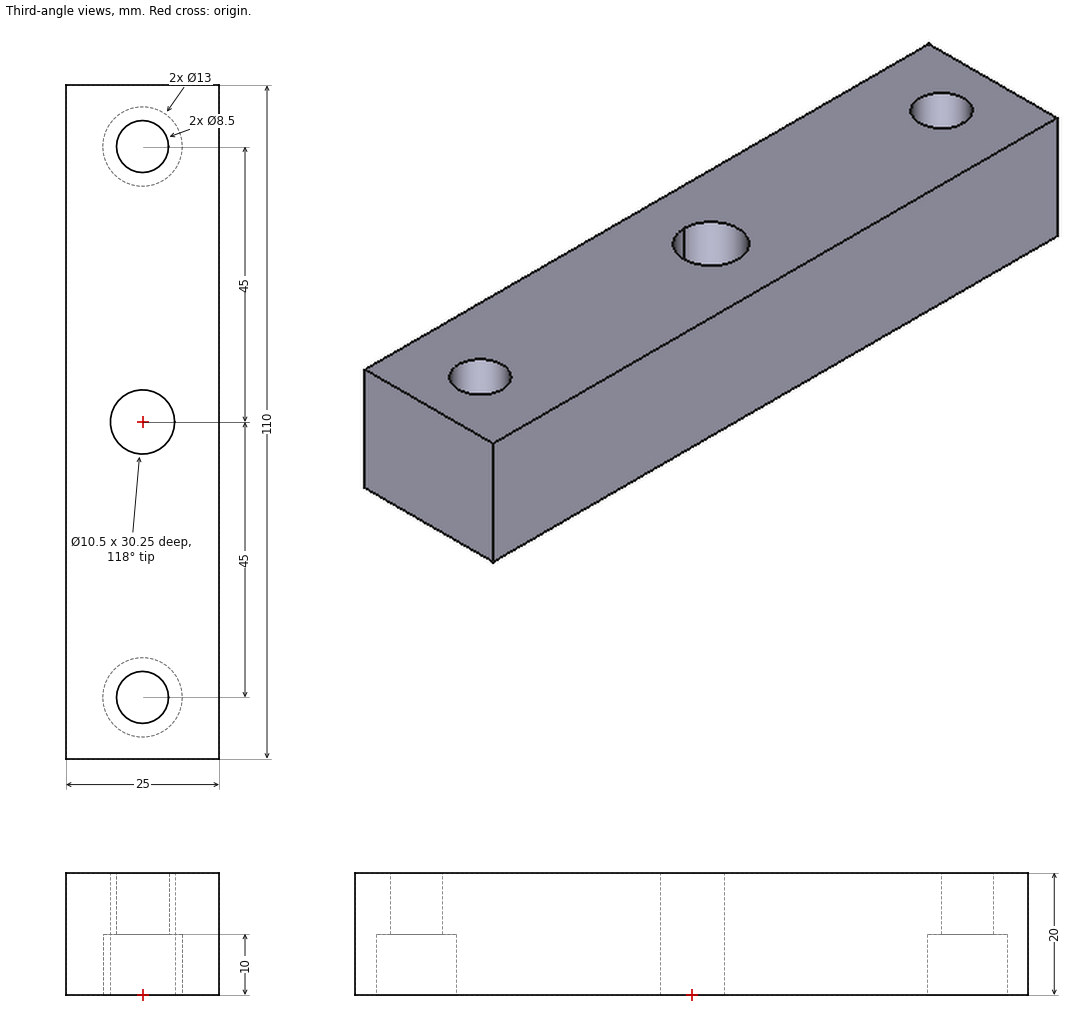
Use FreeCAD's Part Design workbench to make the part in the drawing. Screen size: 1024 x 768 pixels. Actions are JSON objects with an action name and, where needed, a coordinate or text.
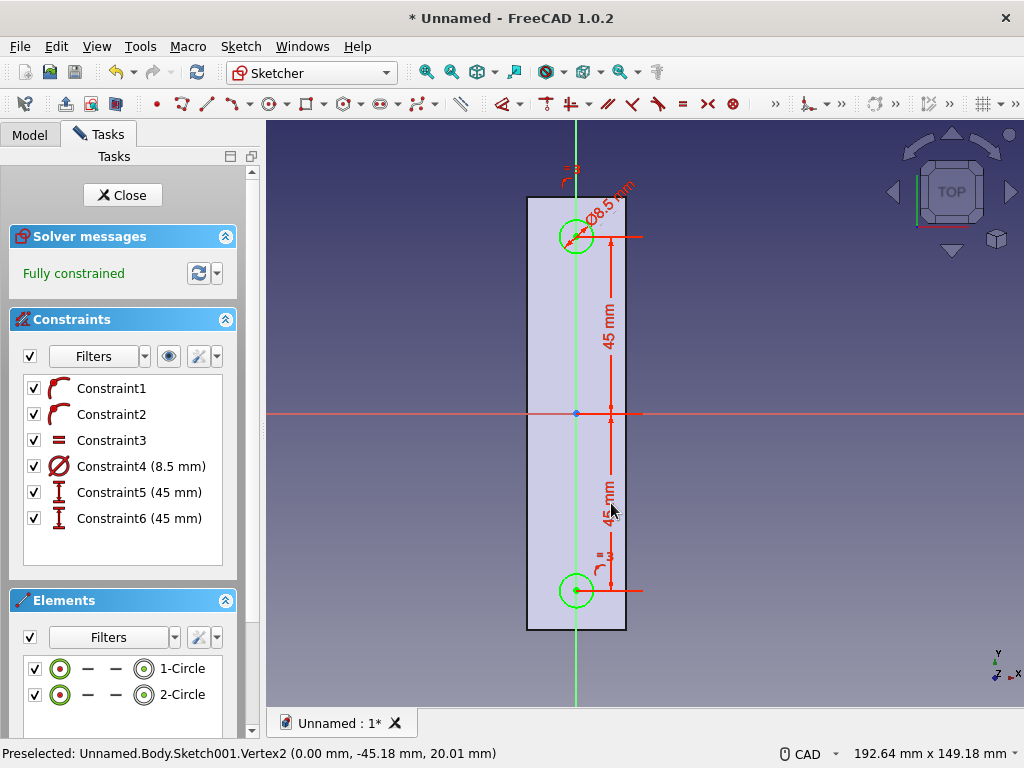
{"action": "left_click", "coordinate": [123, 195]}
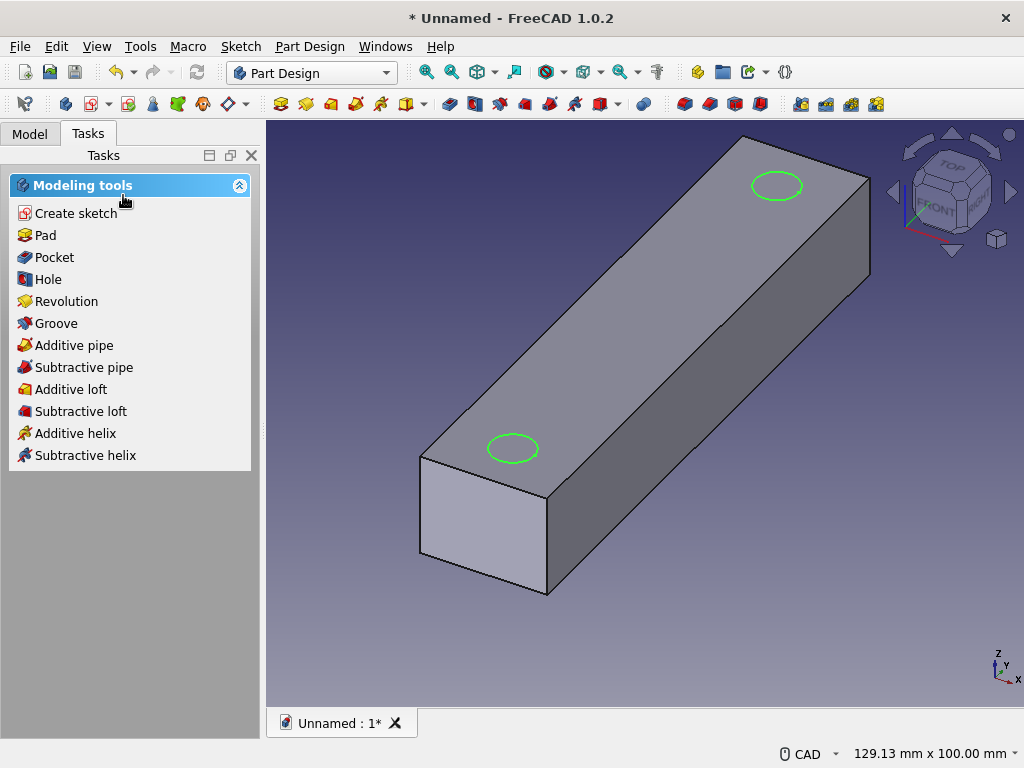
{"action": "left_click", "coordinate": [450, 104]}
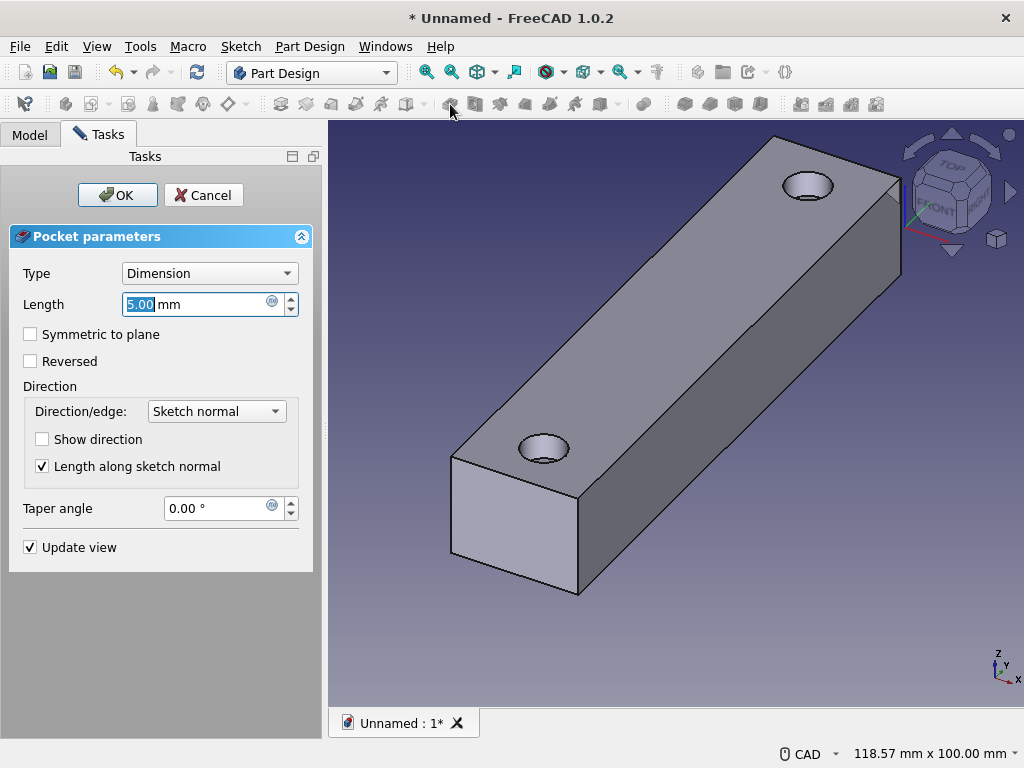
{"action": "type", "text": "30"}
{"action": "key", "text": "Tab"}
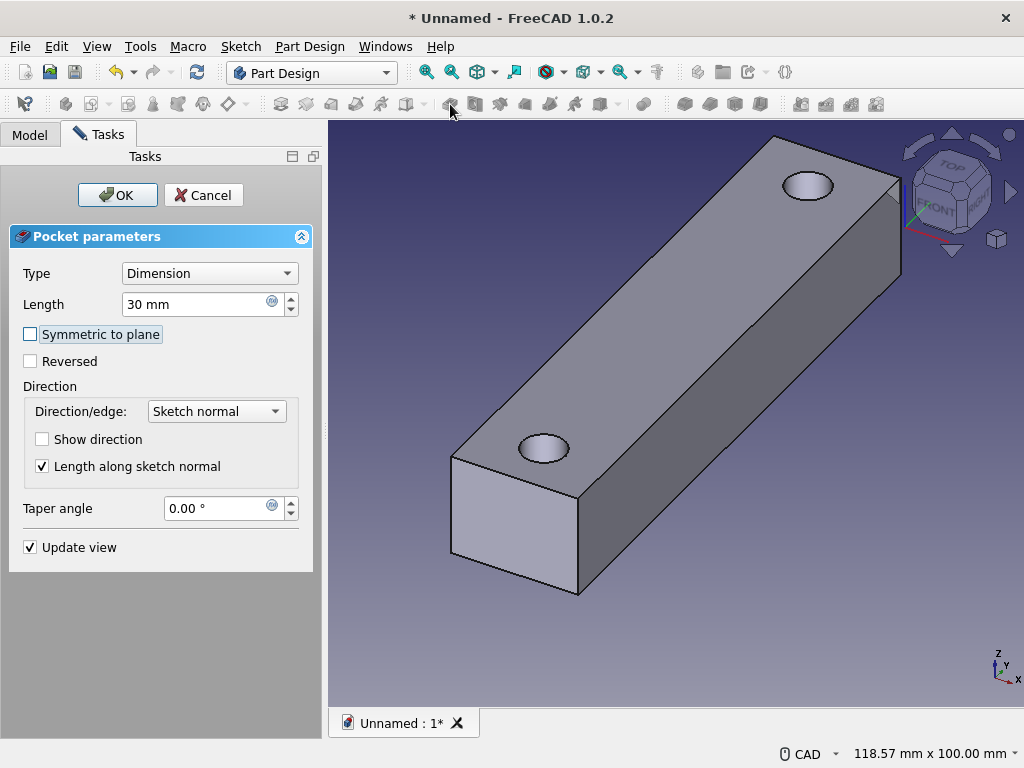
{"action": "left_click", "coordinate": [118, 195]}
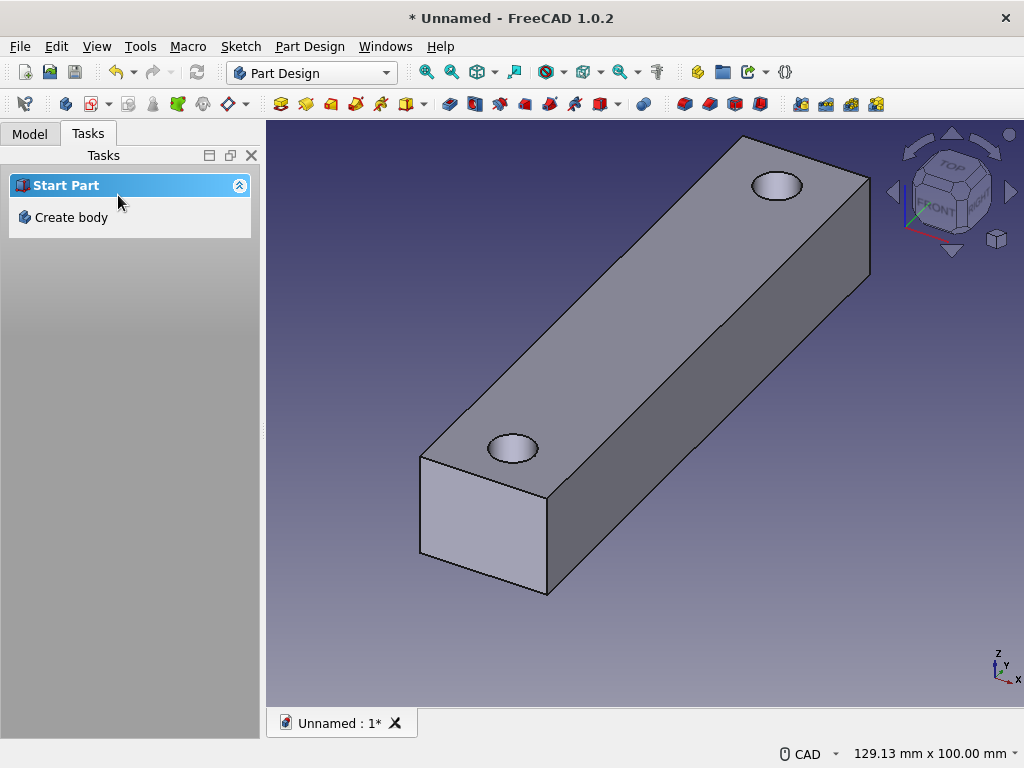
{"action": "key", "text": "5"}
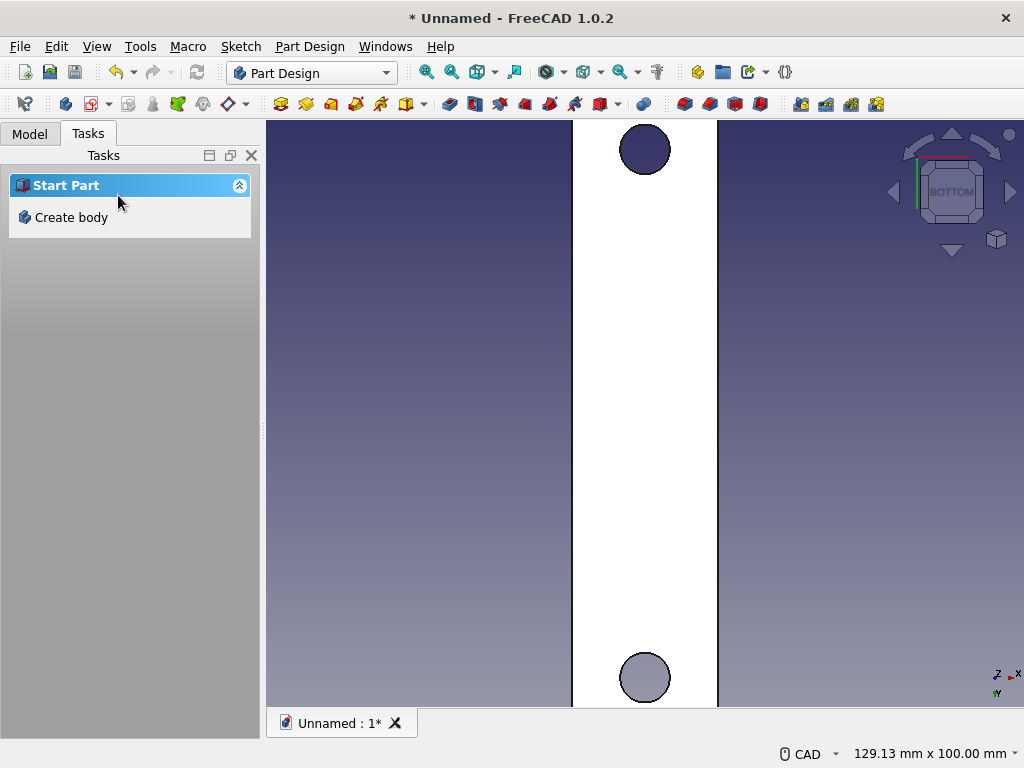
{"action": "left_click", "coordinate": [427, 72]}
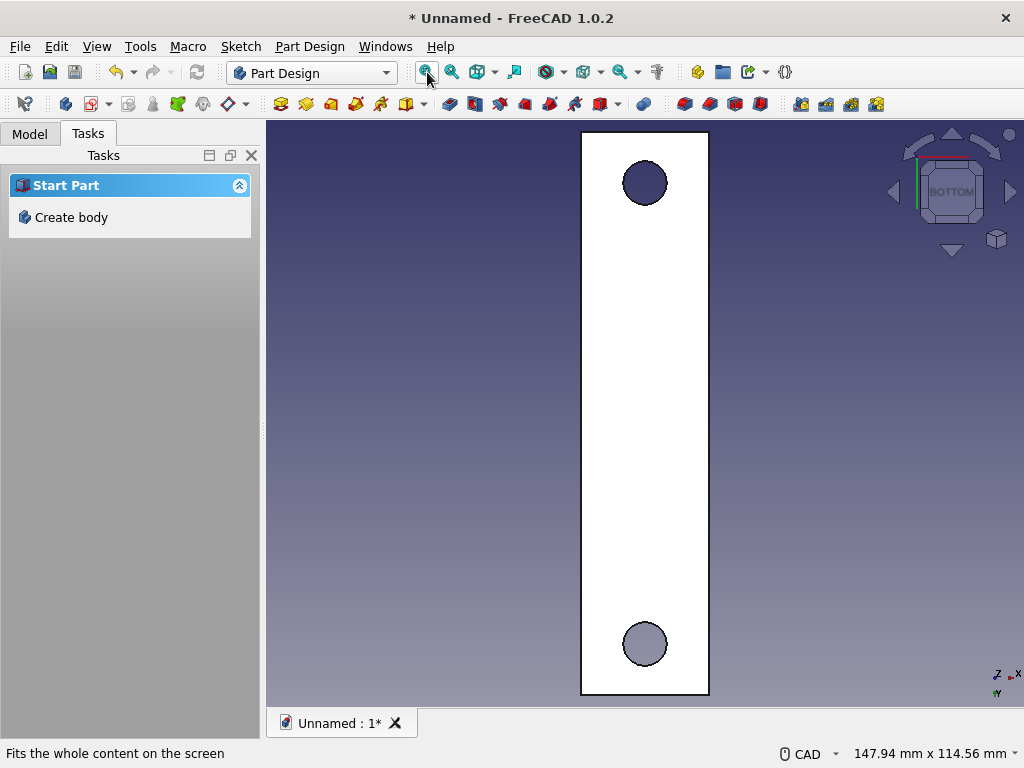
{"action": "left_click", "coordinate": [645, 493]}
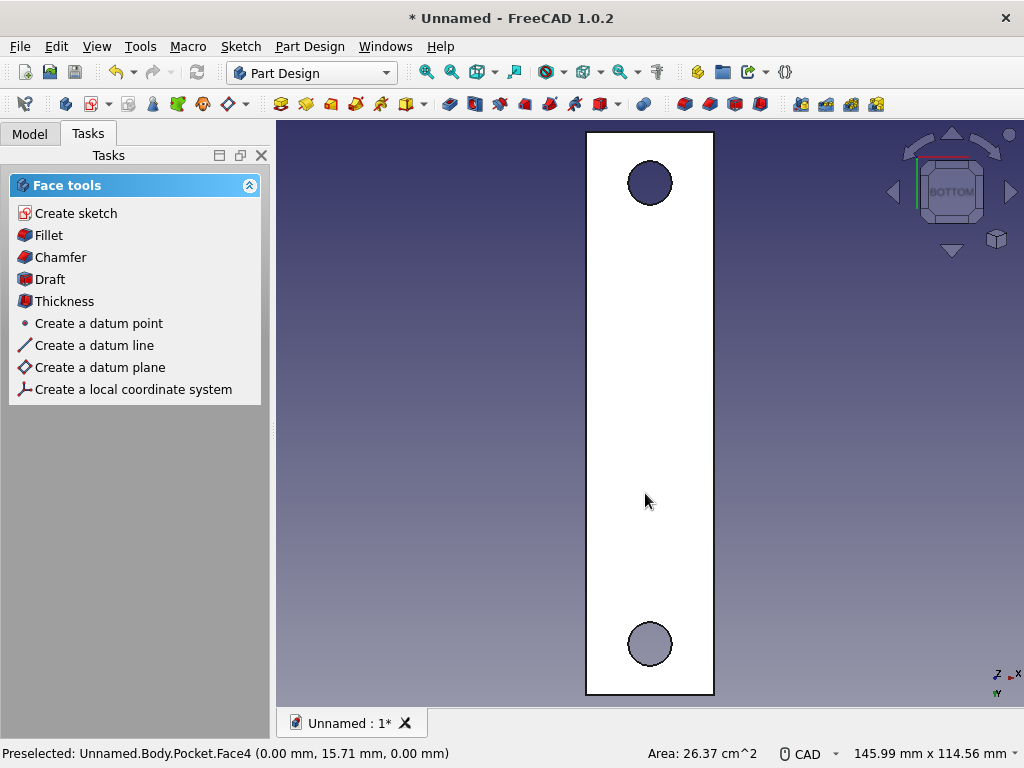
{"action": "left_click", "coordinate": [90, 104]}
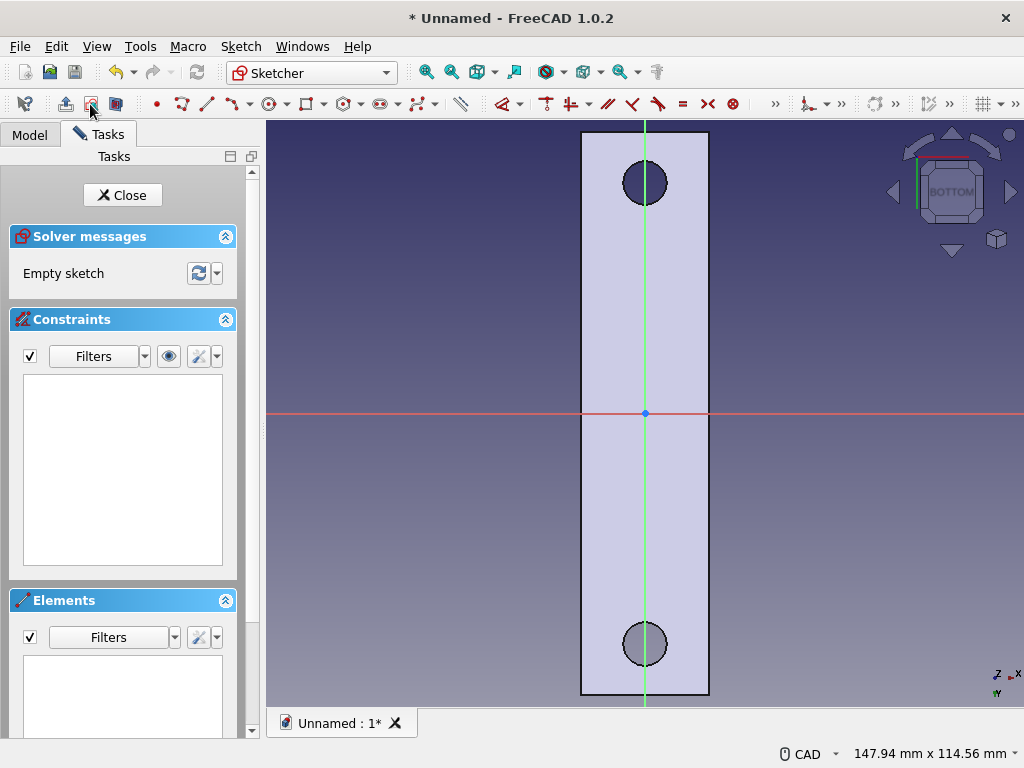
{"action": "scroll", "coordinate": [437, 414], "scroll_direction": "down", "scroll_amount": 2}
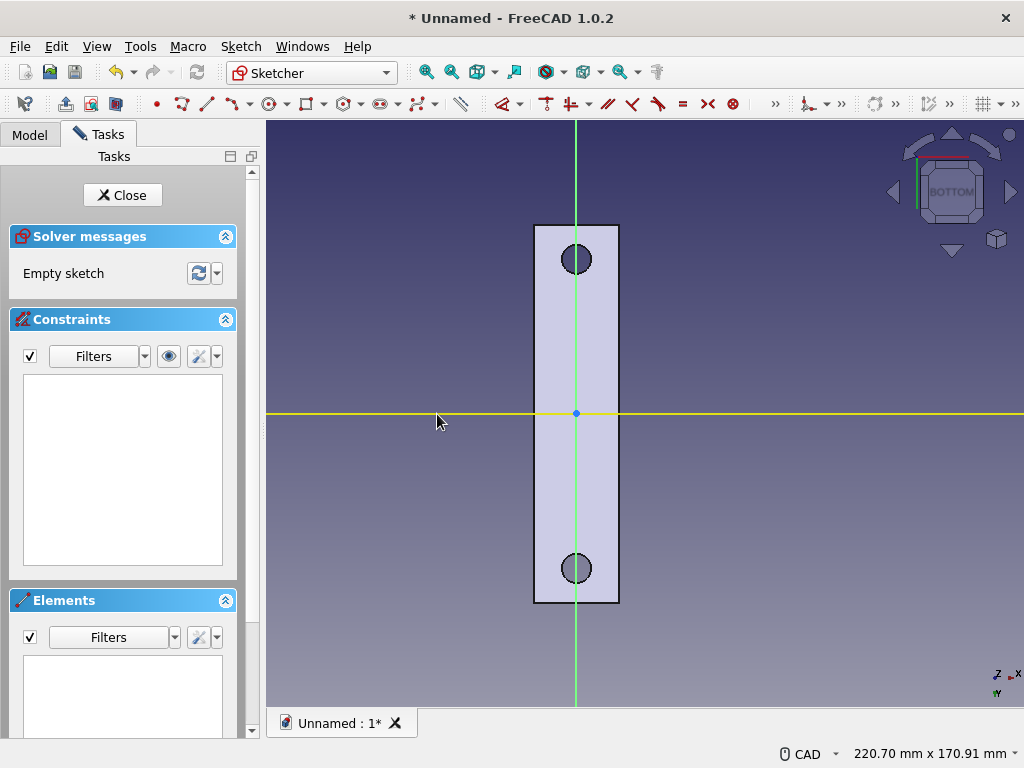
{"action": "key", "text": "g c"}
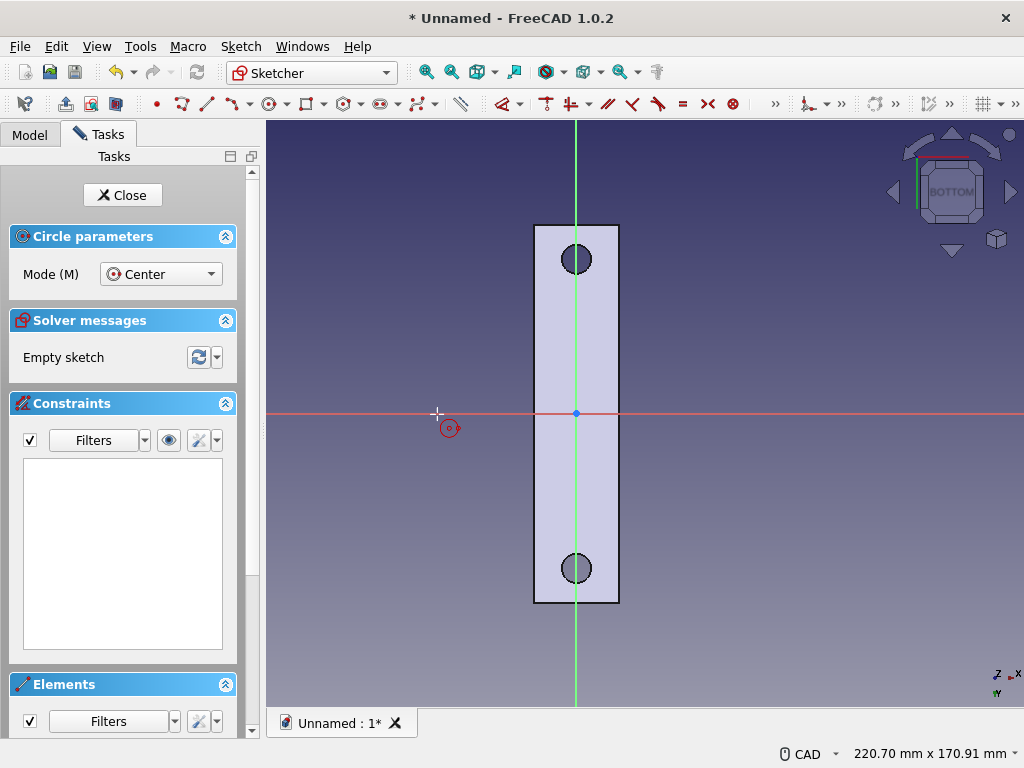
{"action": "left_click", "coordinate": [577, 568]}
{"action": "left_click", "coordinate": [592, 553]}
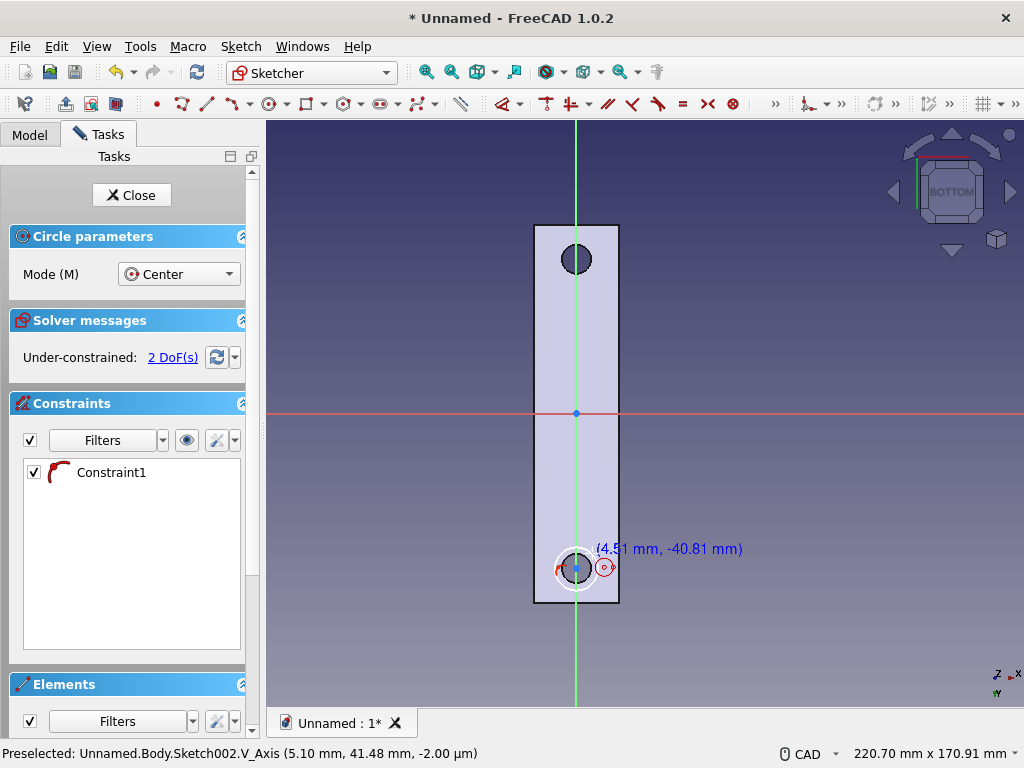
{"action": "left_click", "coordinate": [577, 259]}
{"action": "left_click", "coordinate": [592, 243]}
{"action": "key", "text": "Escape"}